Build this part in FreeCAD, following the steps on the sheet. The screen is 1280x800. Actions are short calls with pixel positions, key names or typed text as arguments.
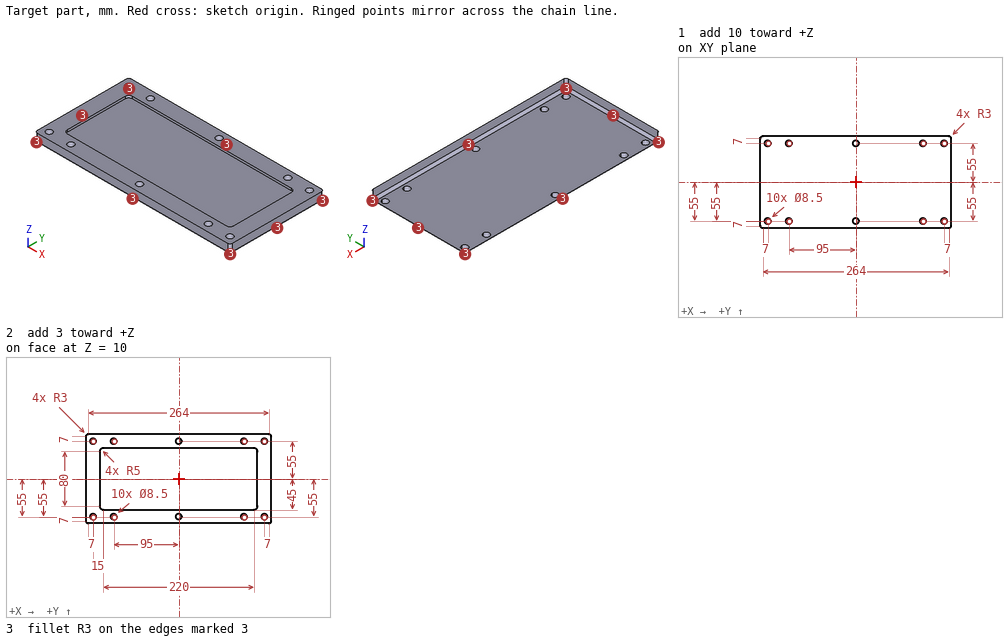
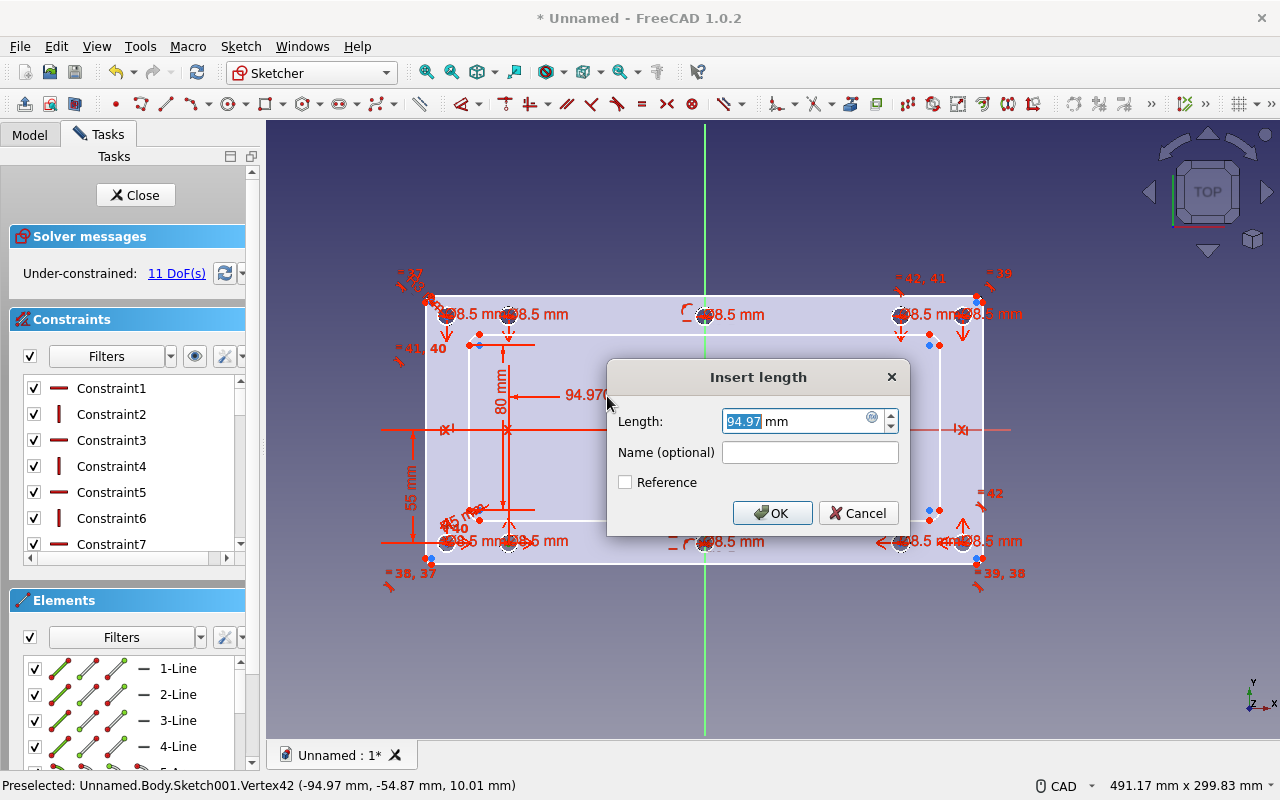
text(95)
key(Return)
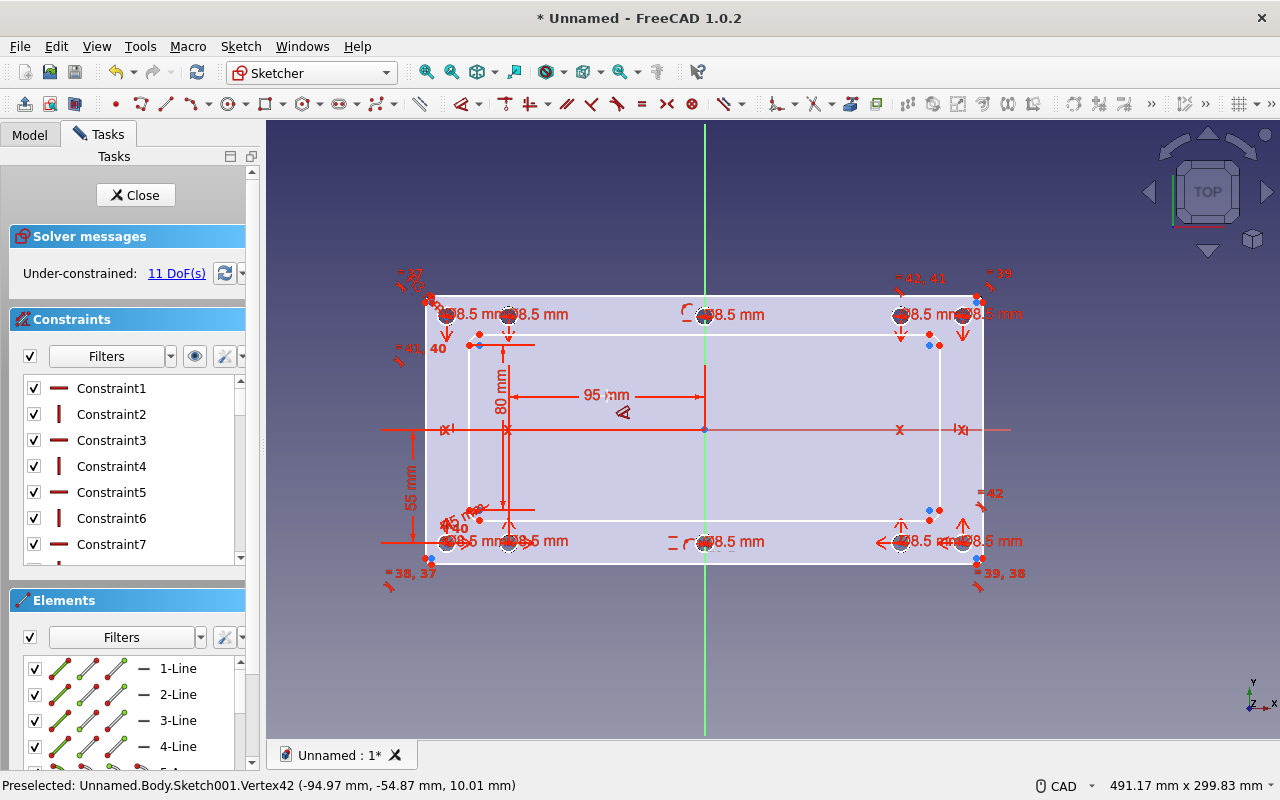
click(509, 543)
click(739, 486)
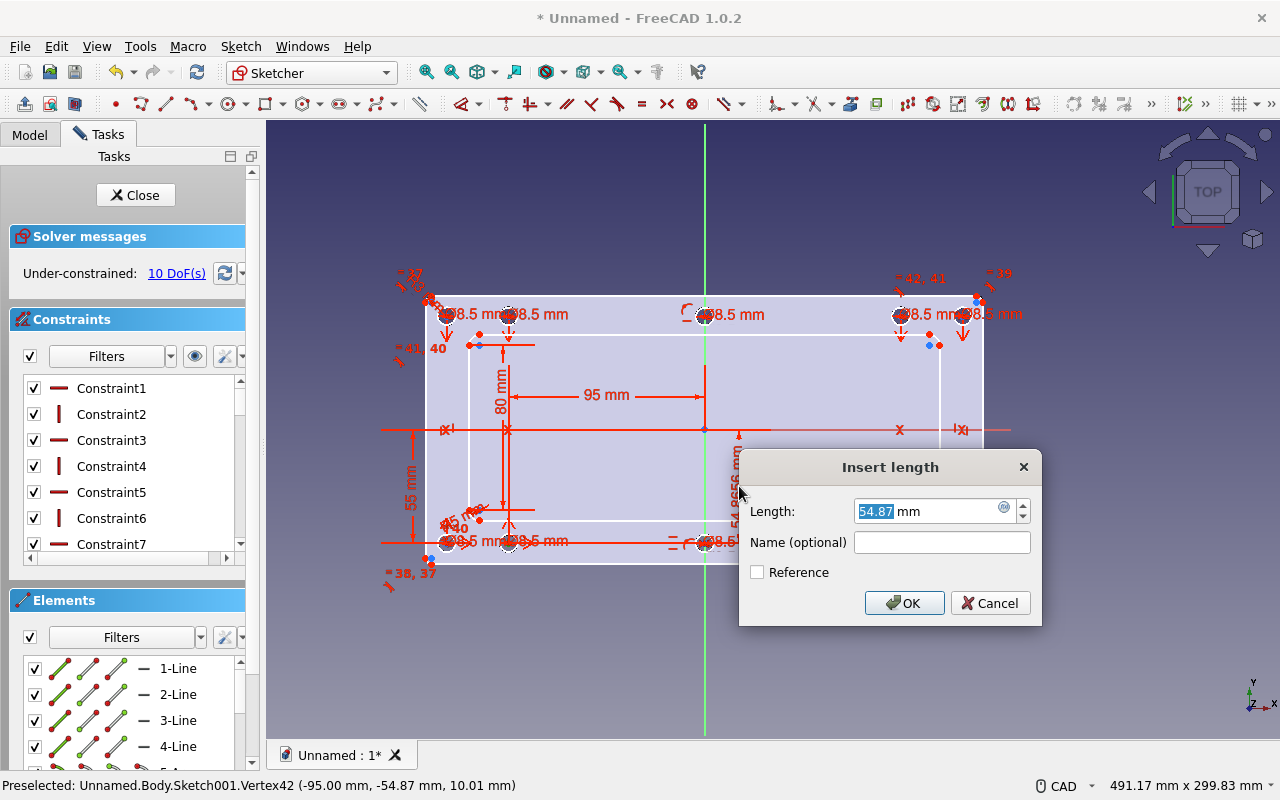
text(55)
key(Return)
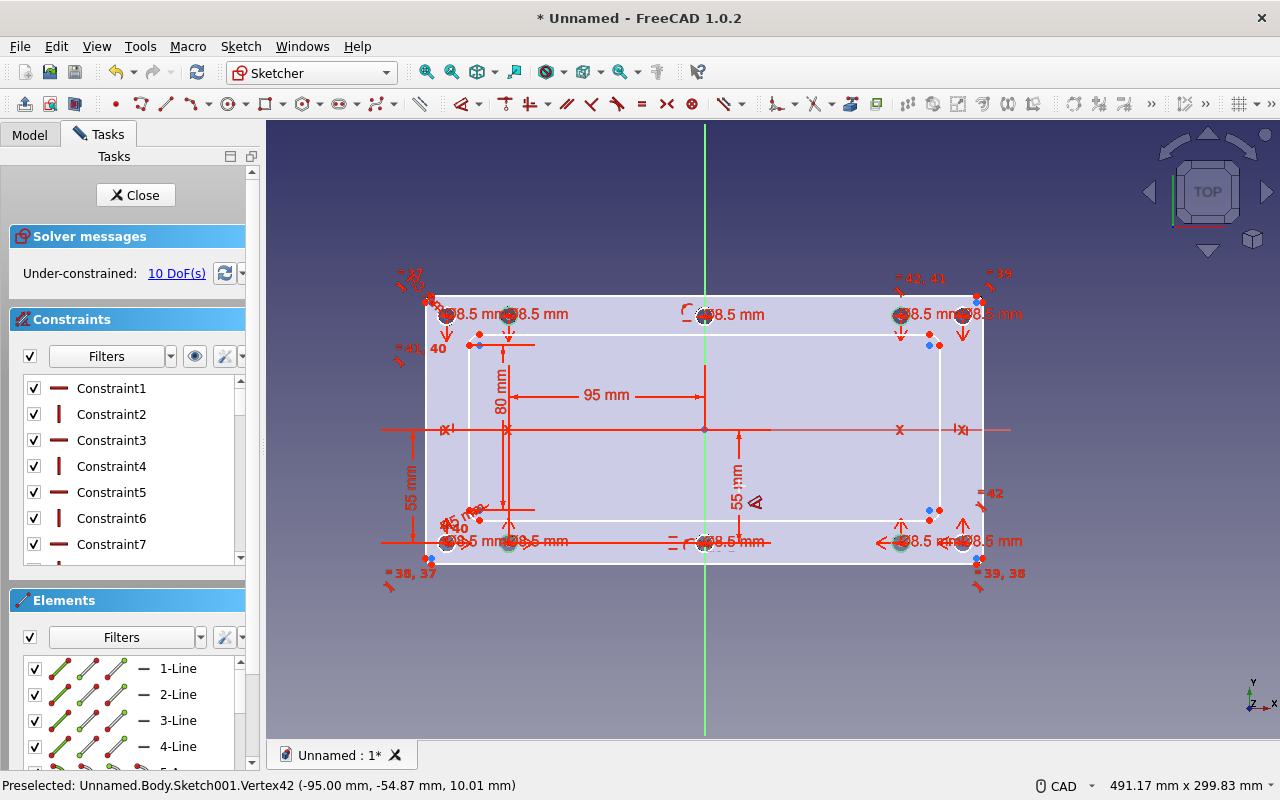
click(705, 544)
click(739, 460)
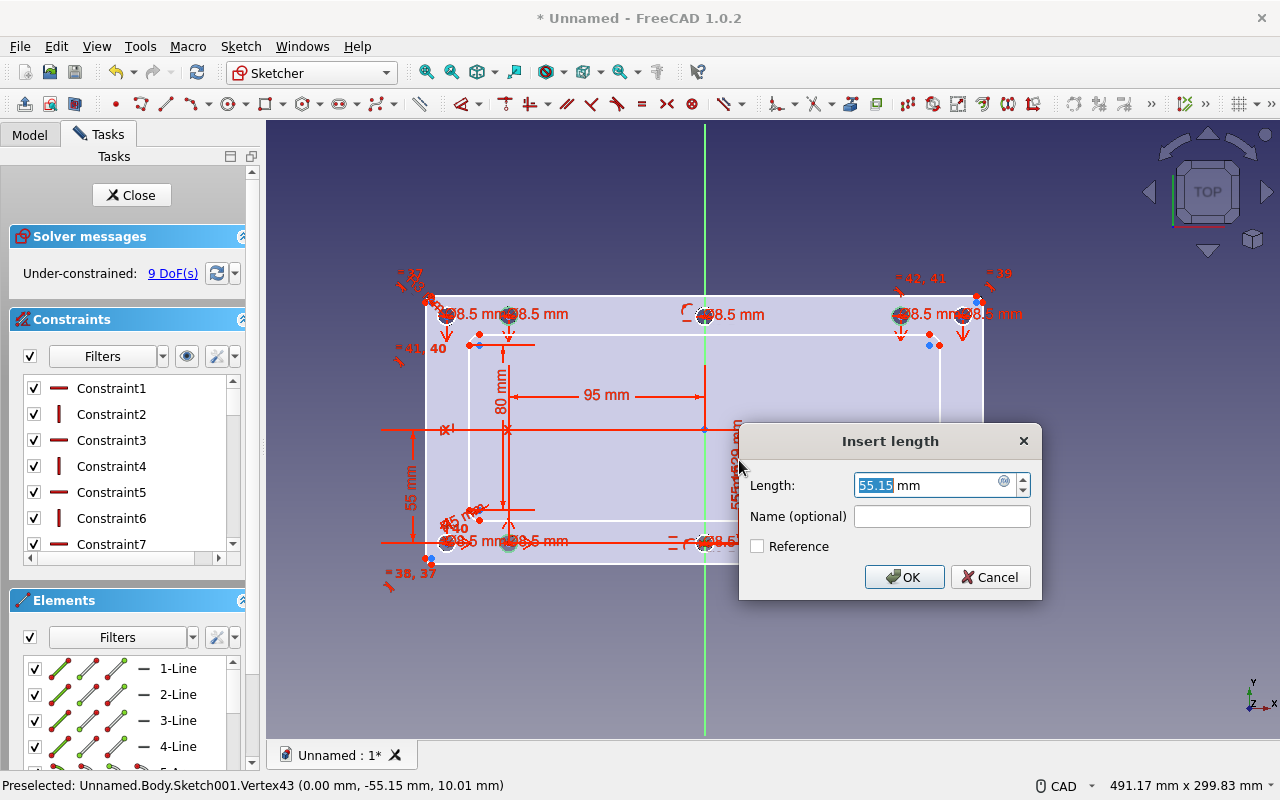
text(55)
key(Return)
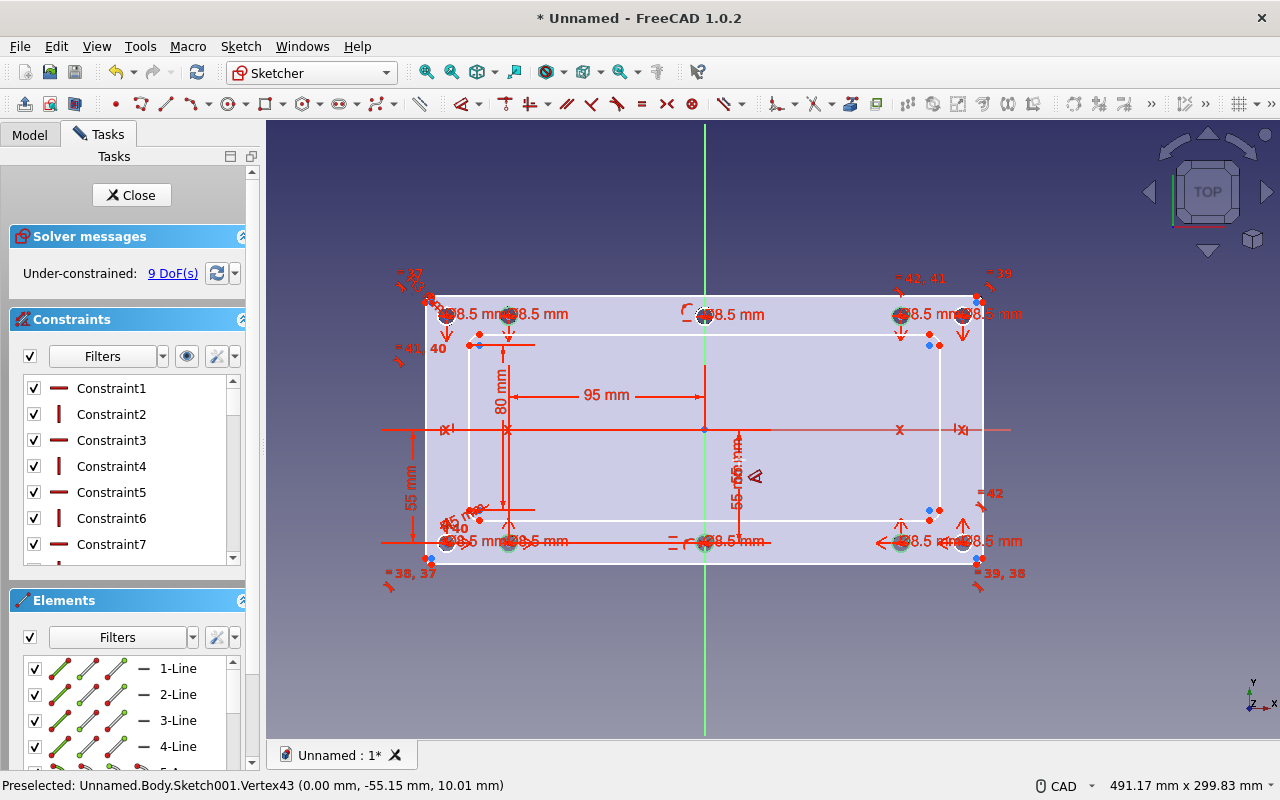
click(705, 317)
click(739, 373)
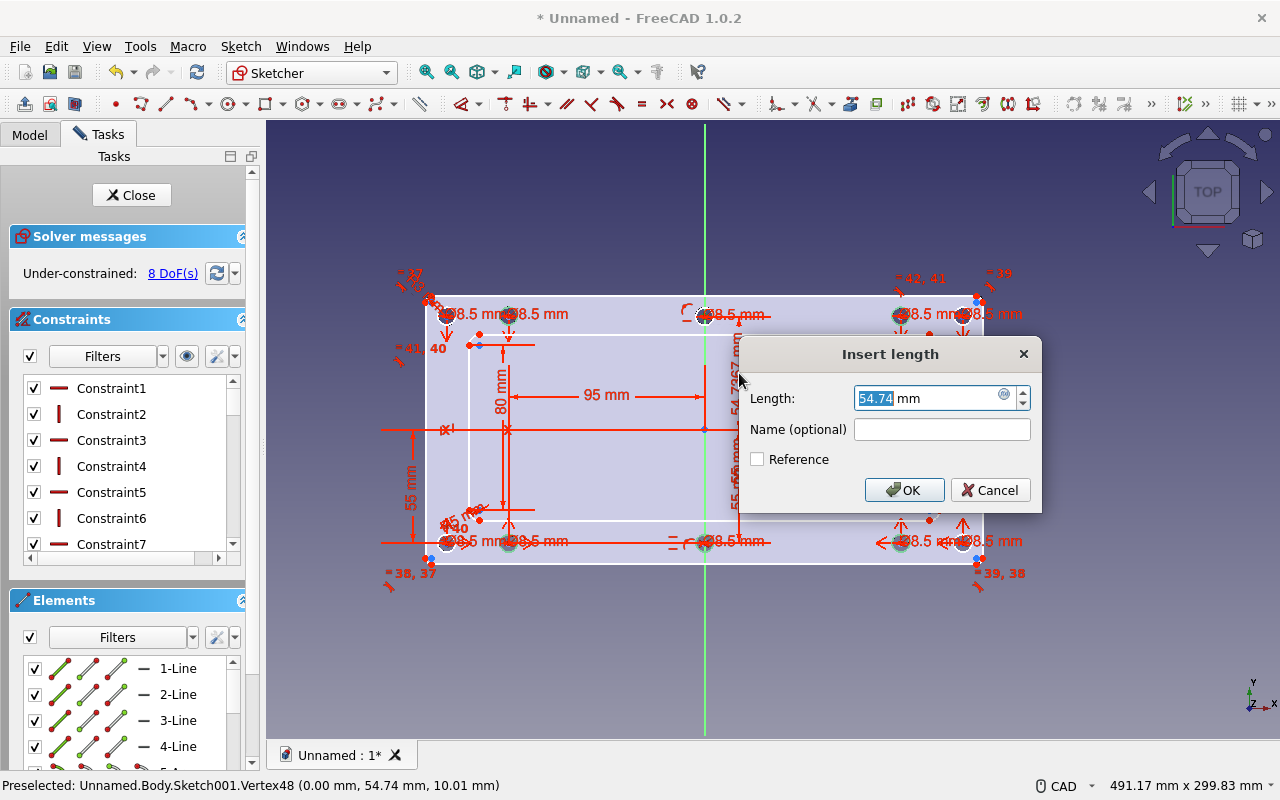
text(55)
key(Return)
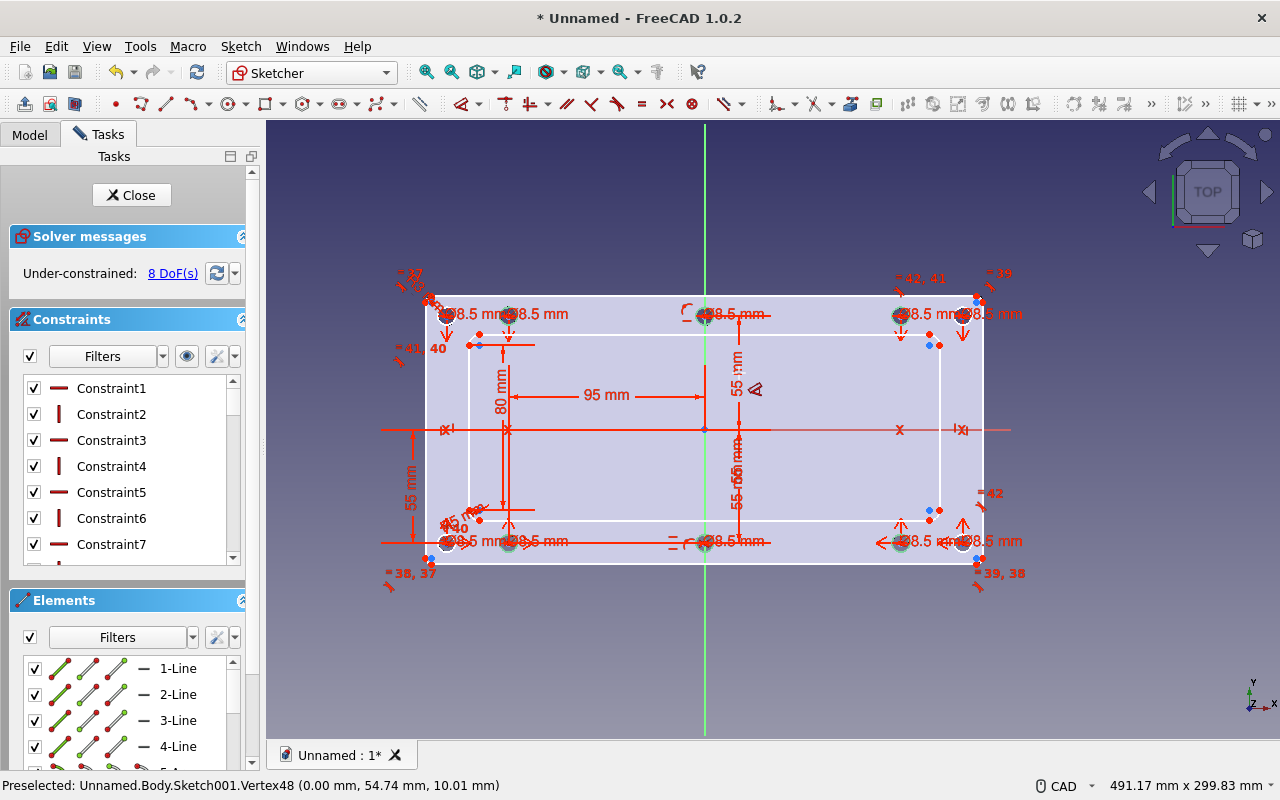
scroll(432, 564, up, 6)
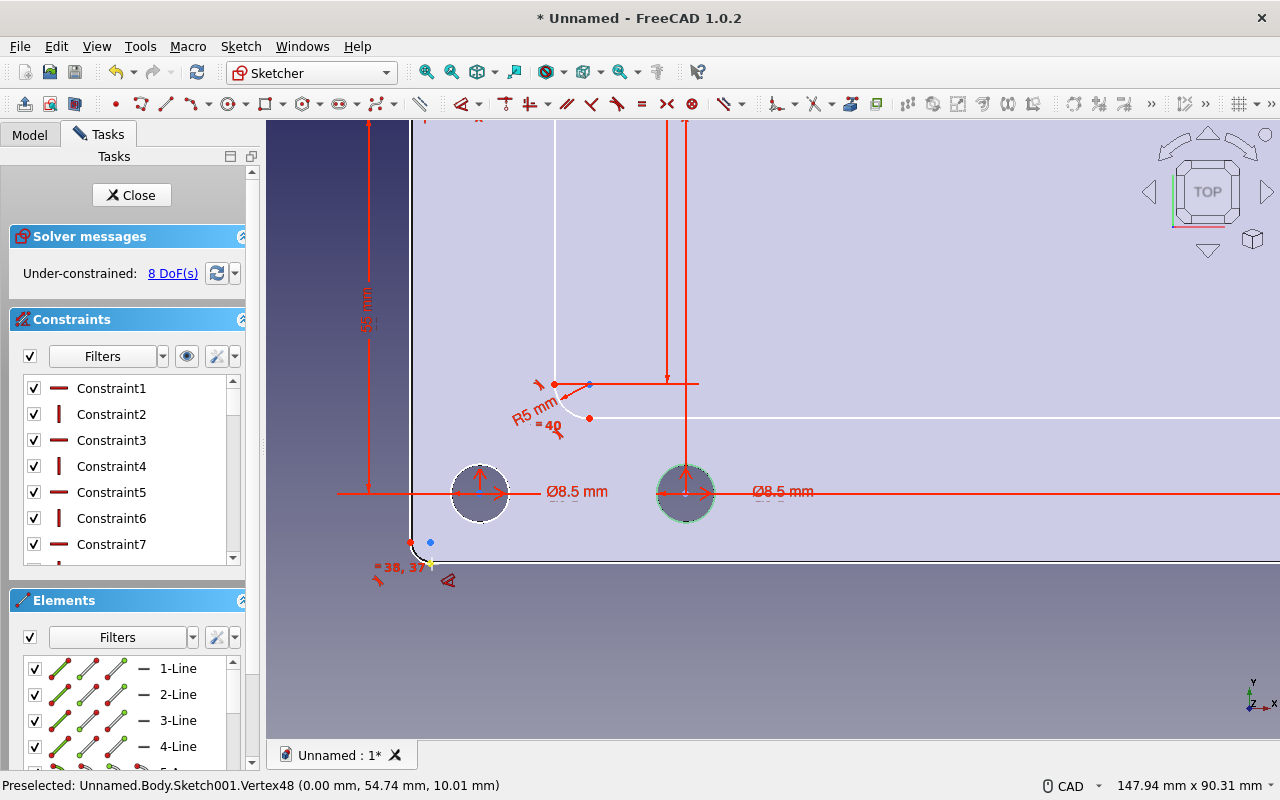
click(431, 563)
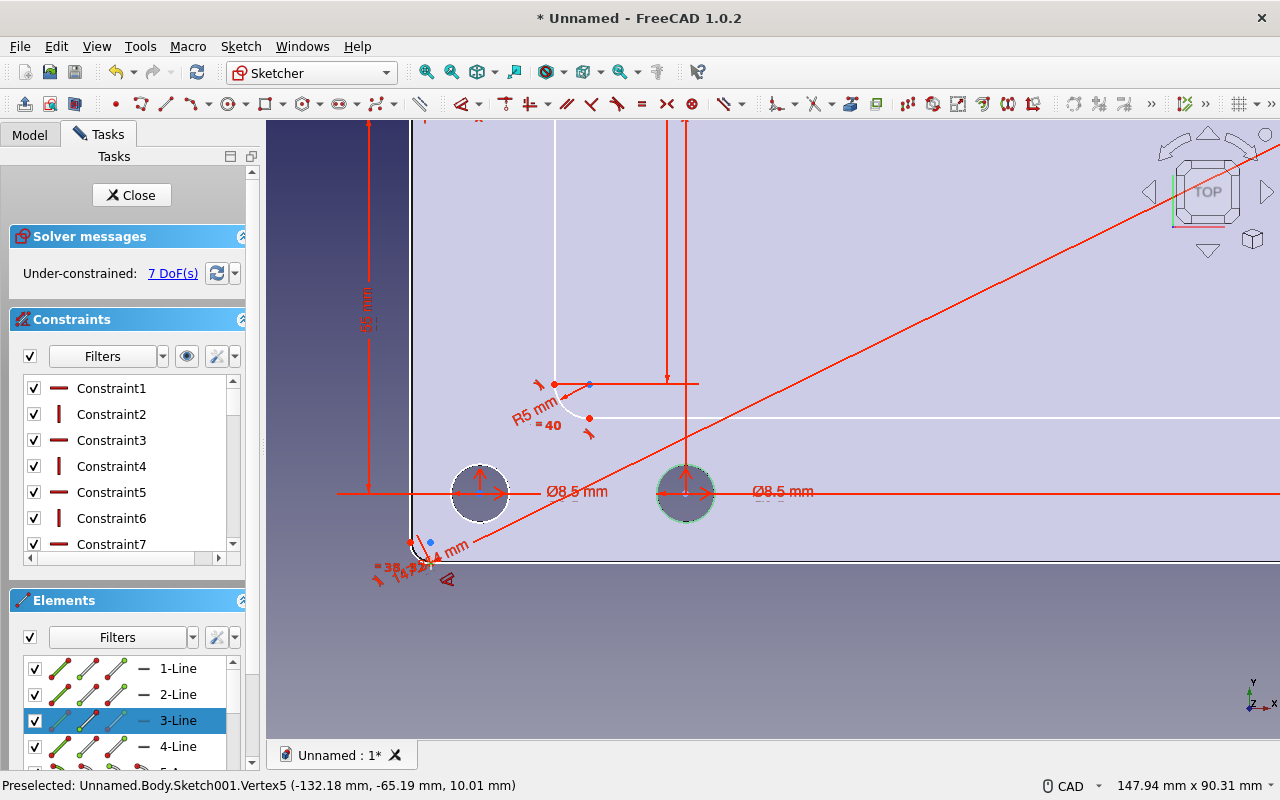
click(480, 494)
click(455, 597)